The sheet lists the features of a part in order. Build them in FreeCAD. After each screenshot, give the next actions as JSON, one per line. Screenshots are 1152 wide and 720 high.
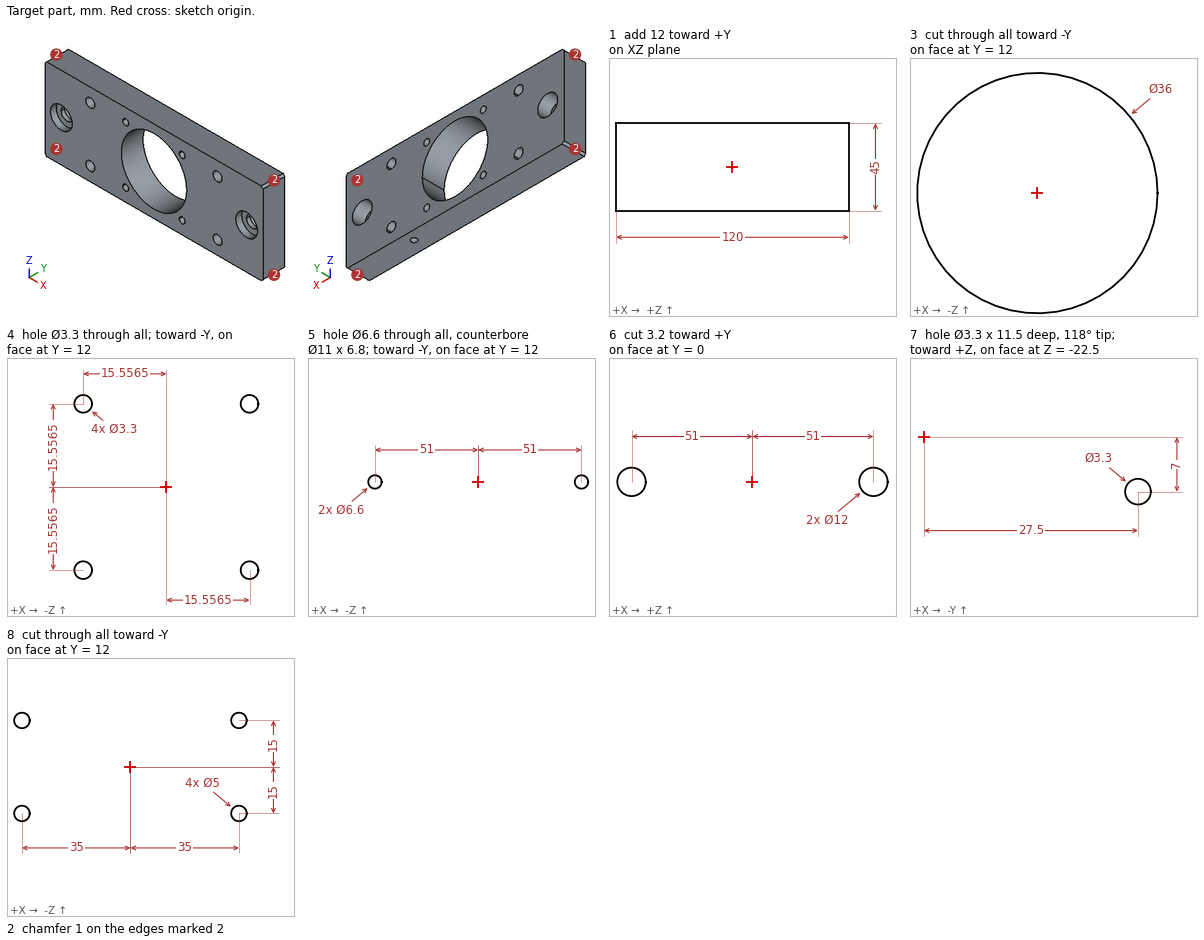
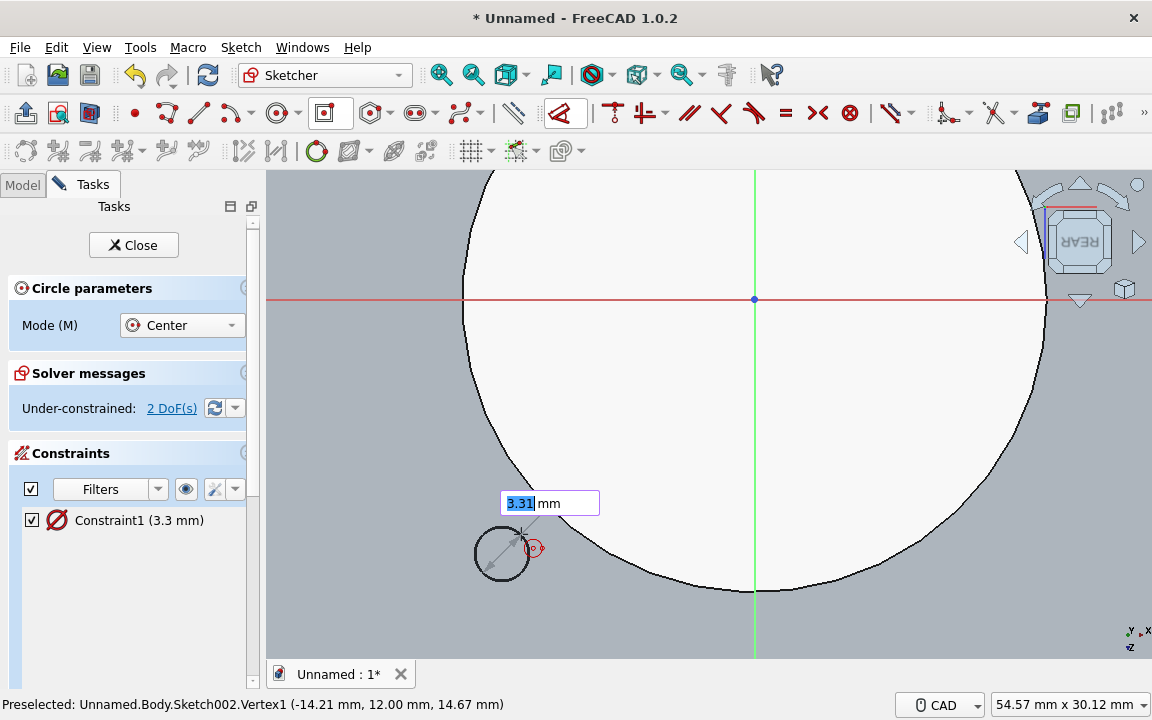
{"action": "type", "text": "3.3"}
{"action": "key", "text": "Return"}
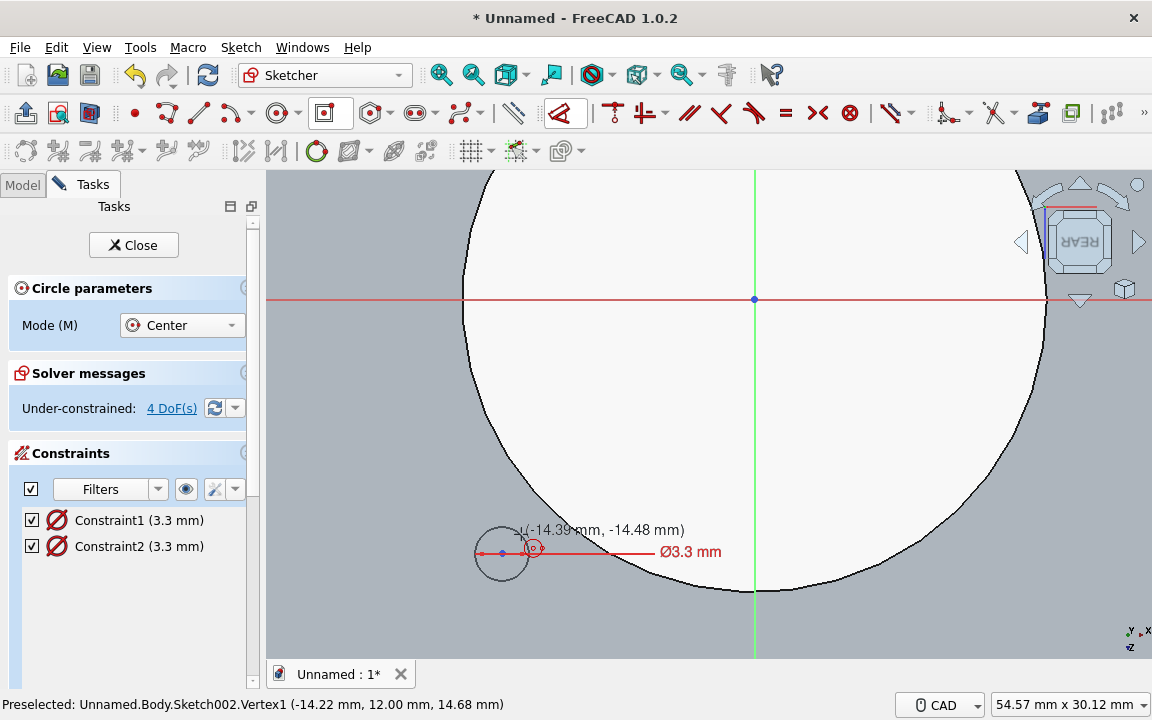
{"action": "scroll", "coordinate": [502, 554], "scroll_direction": "down", "scroll_amount": 3}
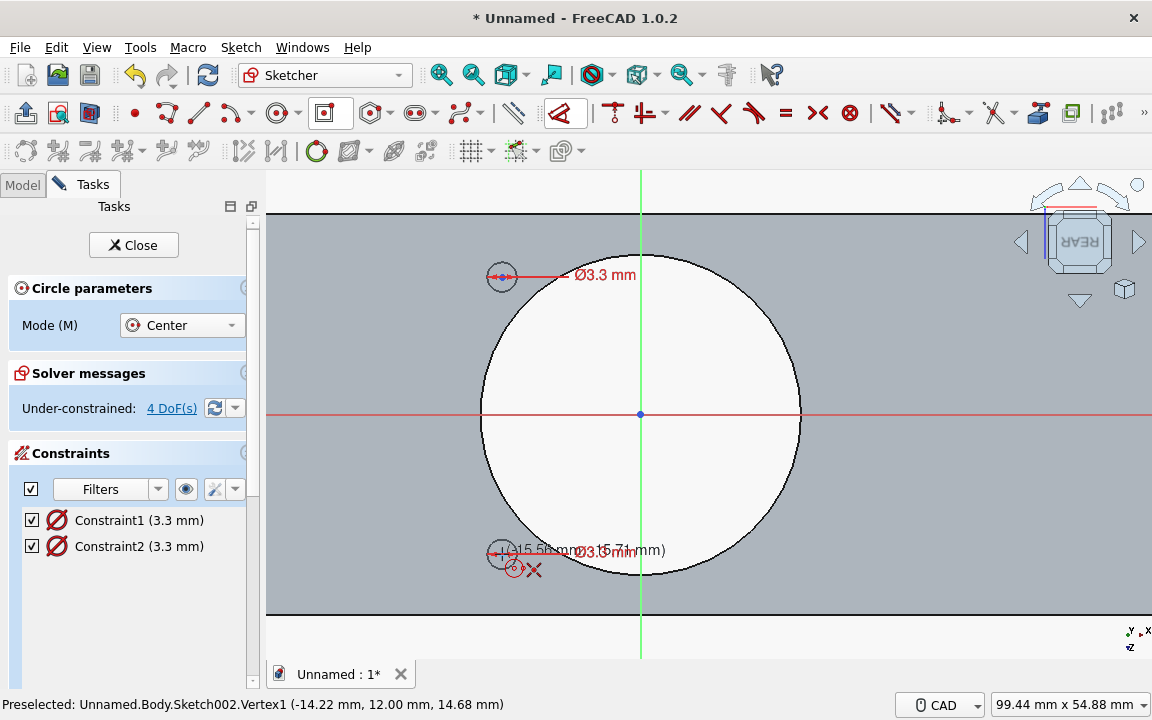
{"action": "scroll", "coordinate": [779, 554], "scroll_direction": "up", "scroll_amount": 3}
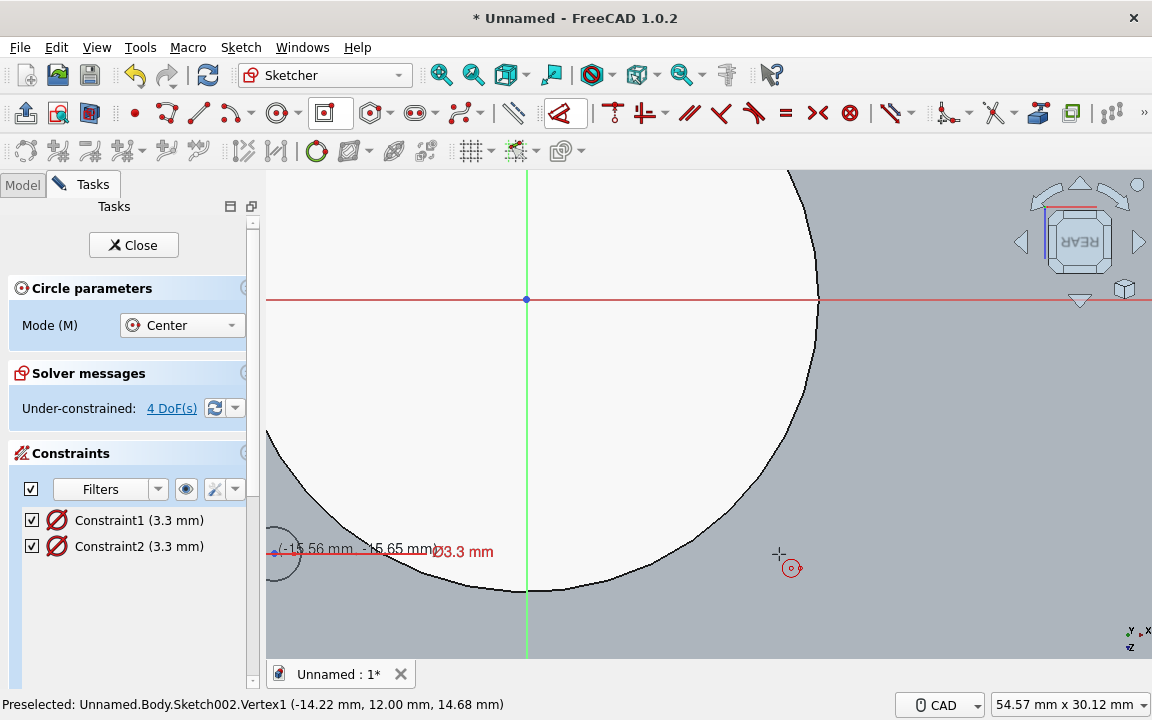
{"action": "left_click", "coordinate": [779, 553]}
{"action": "mouse_move", "coordinate": [798, 534]}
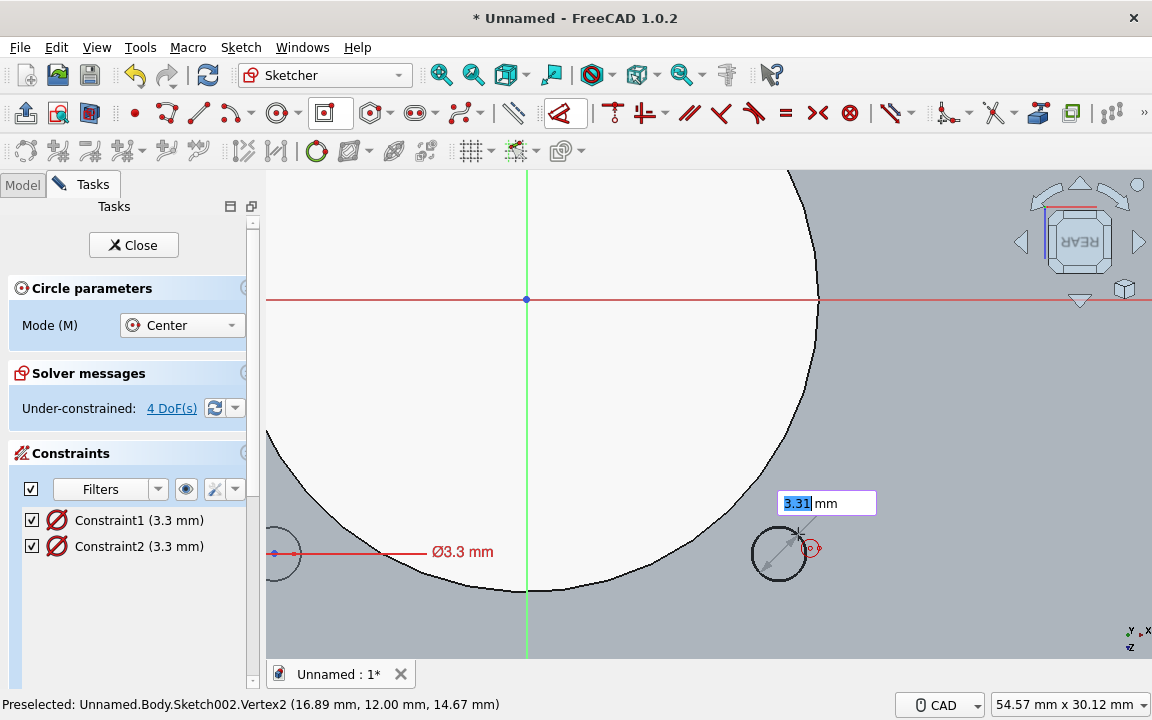
{"action": "type", "text": "3.3"}
{"action": "key", "text": "Return"}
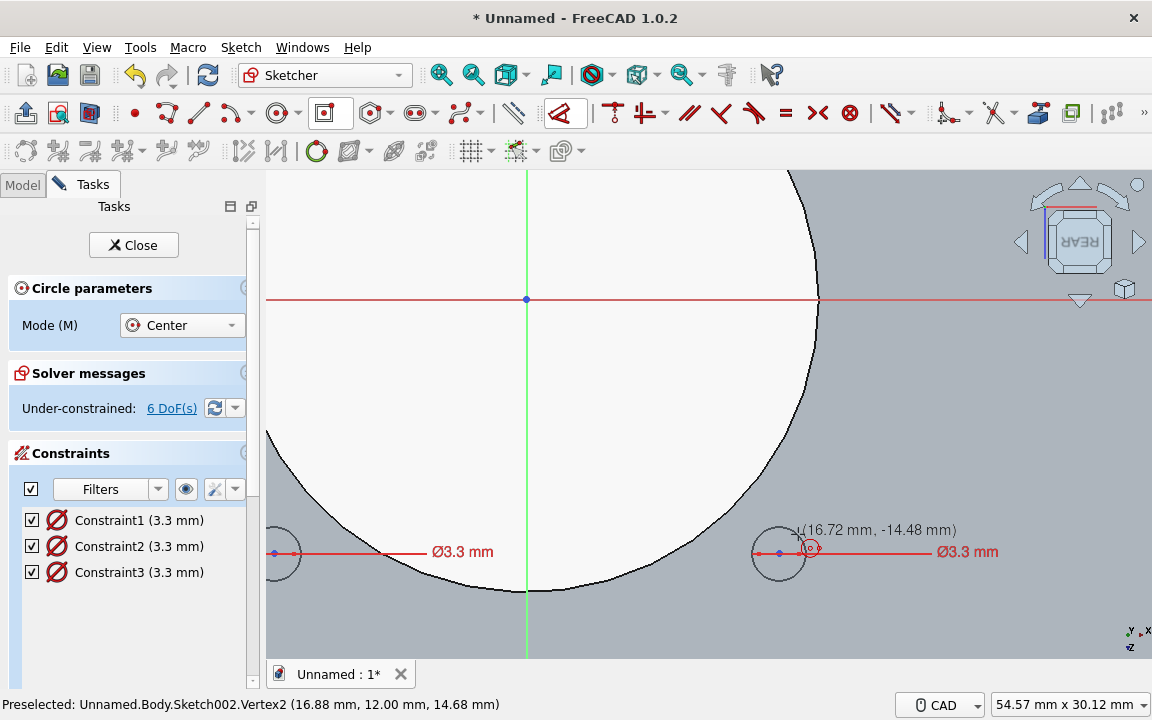
{"action": "scroll", "coordinate": [779, 554], "scroll_direction": "down", "scroll_amount": 3}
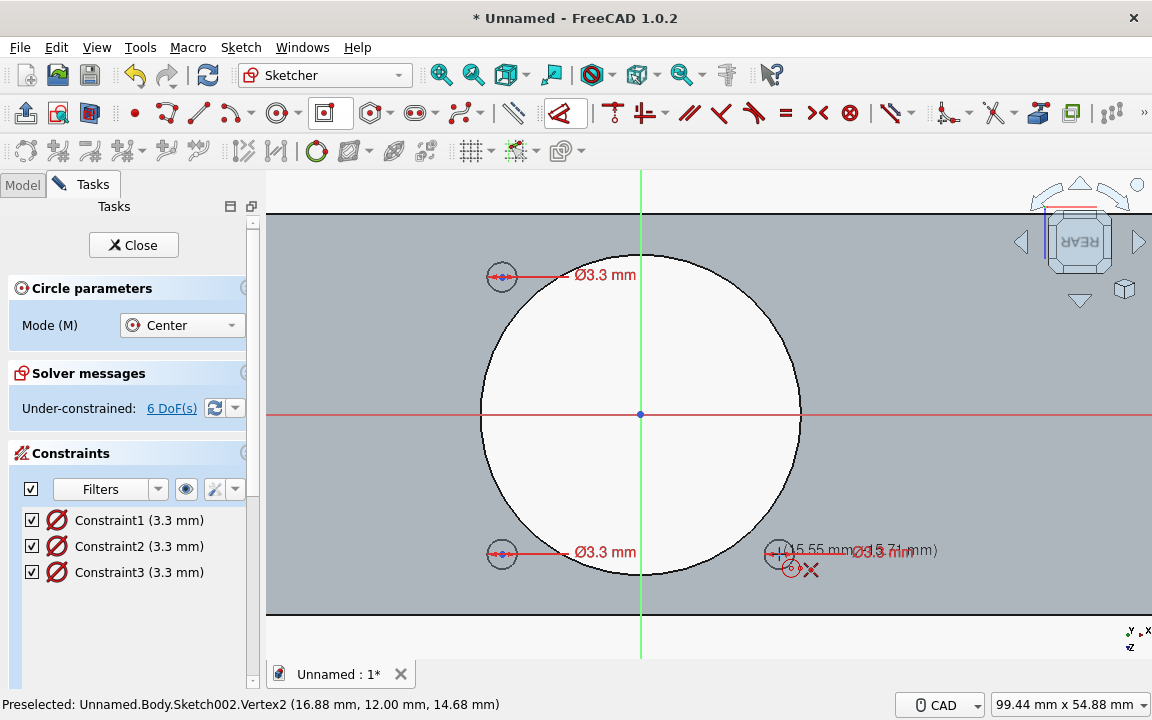
{"action": "scroll", "coordinate": [779, 276], "scroll_direction": "up", "scroll_amount": 3}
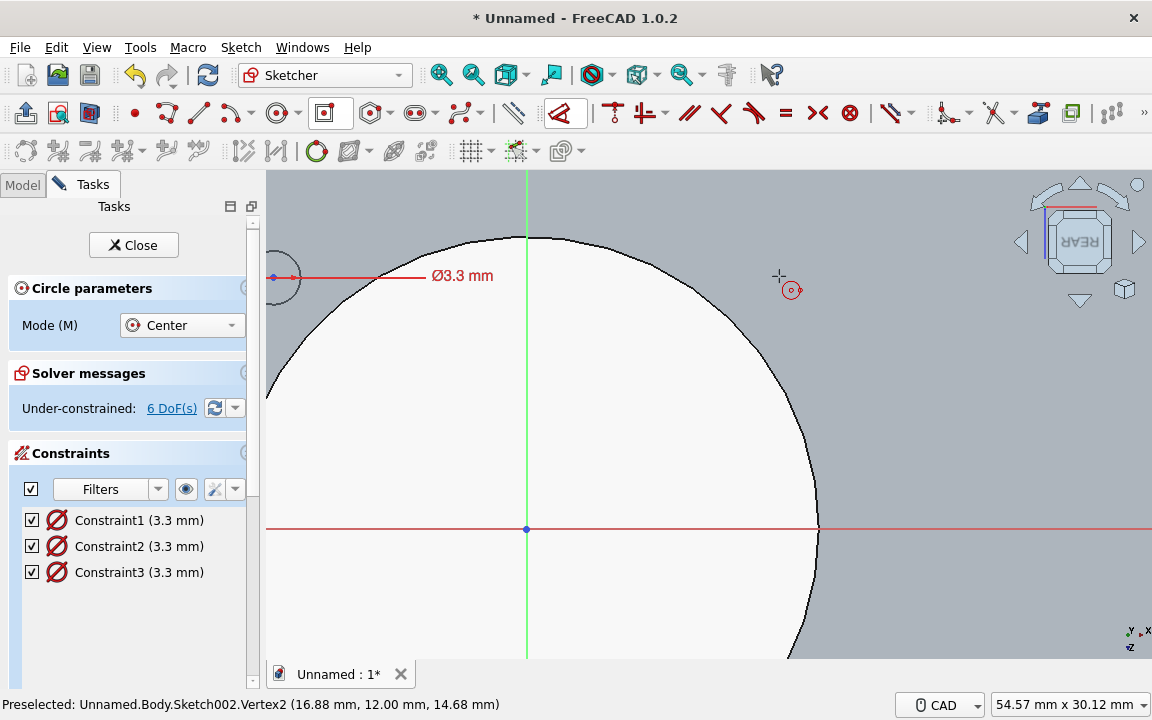
{"action": "left_click", "coordinate": [779, 276]}
{"action": "mouse_move", "coordinate": [798, 258]}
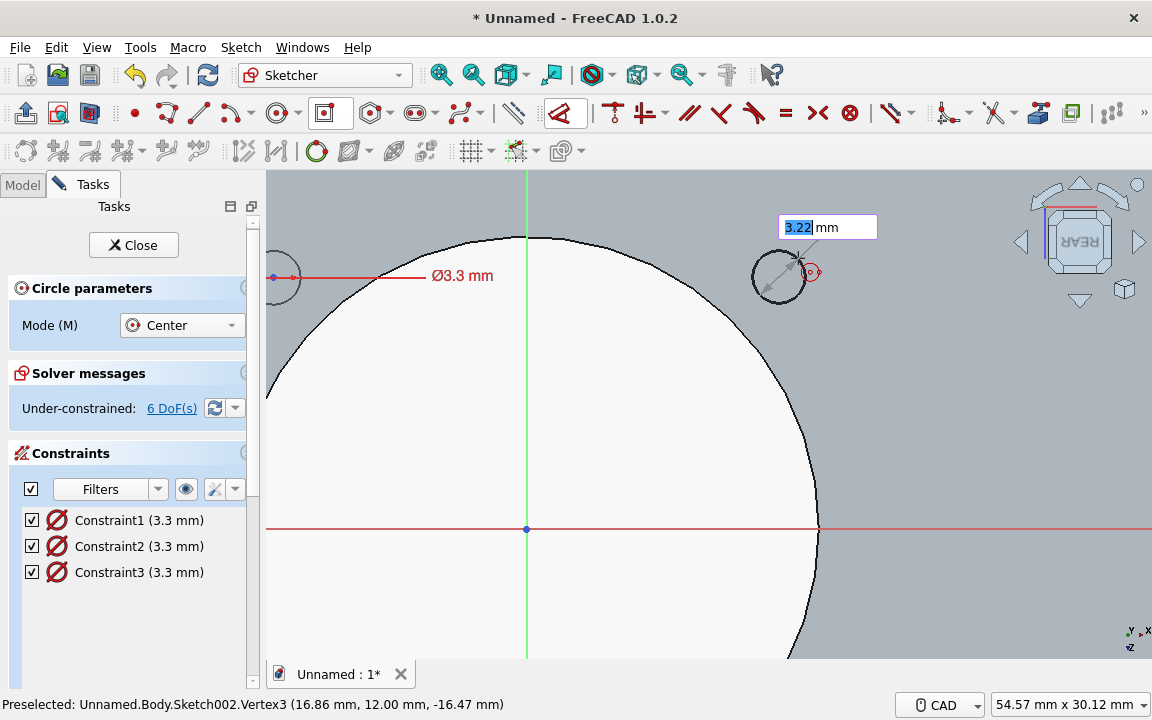
{"action": "type", "text": "3.3"}
{"action": "key", "text": "Return"}
{"action": "key", "text": "Escape"}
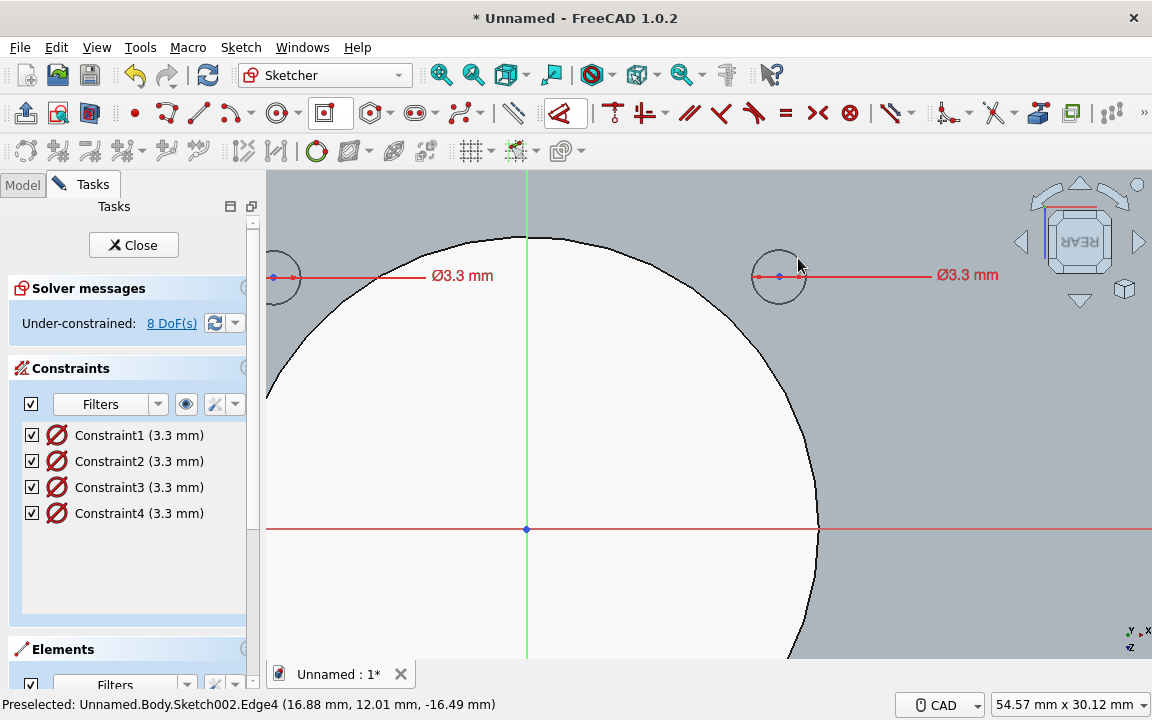
{"action": "scroll", "coordinate": [779, 275], "scroll_direction": "down", "scroll_amount": 3}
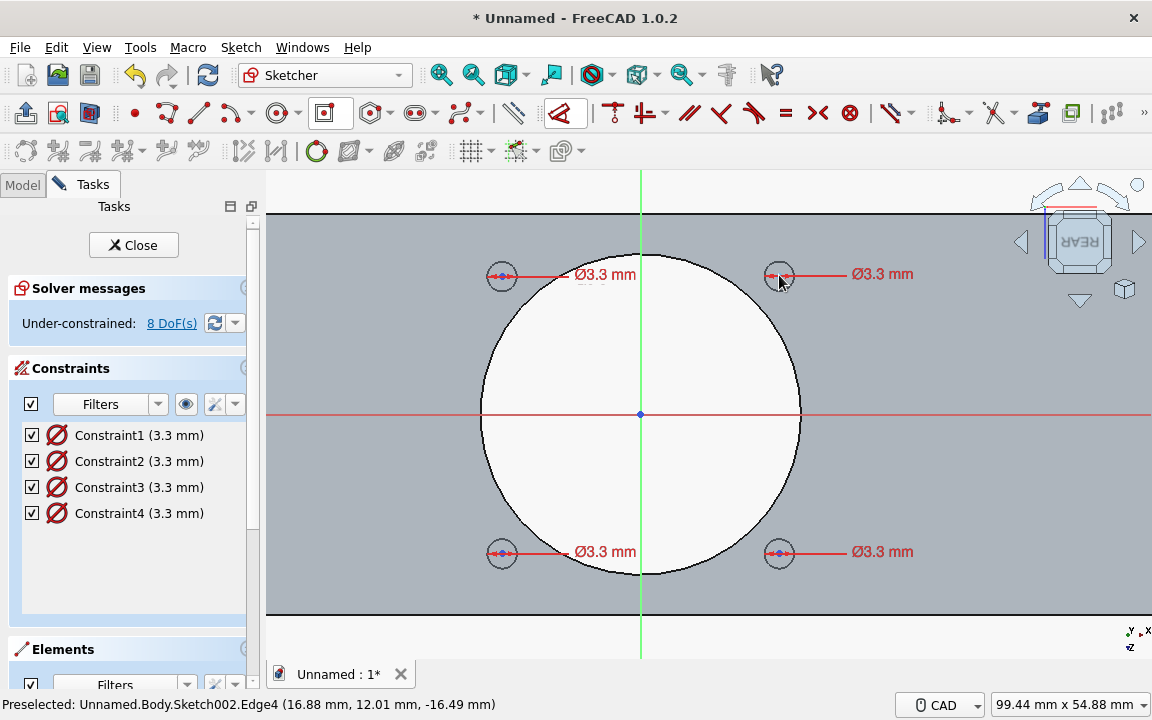
{"action": "left_click", "coordinate": [502, 277]}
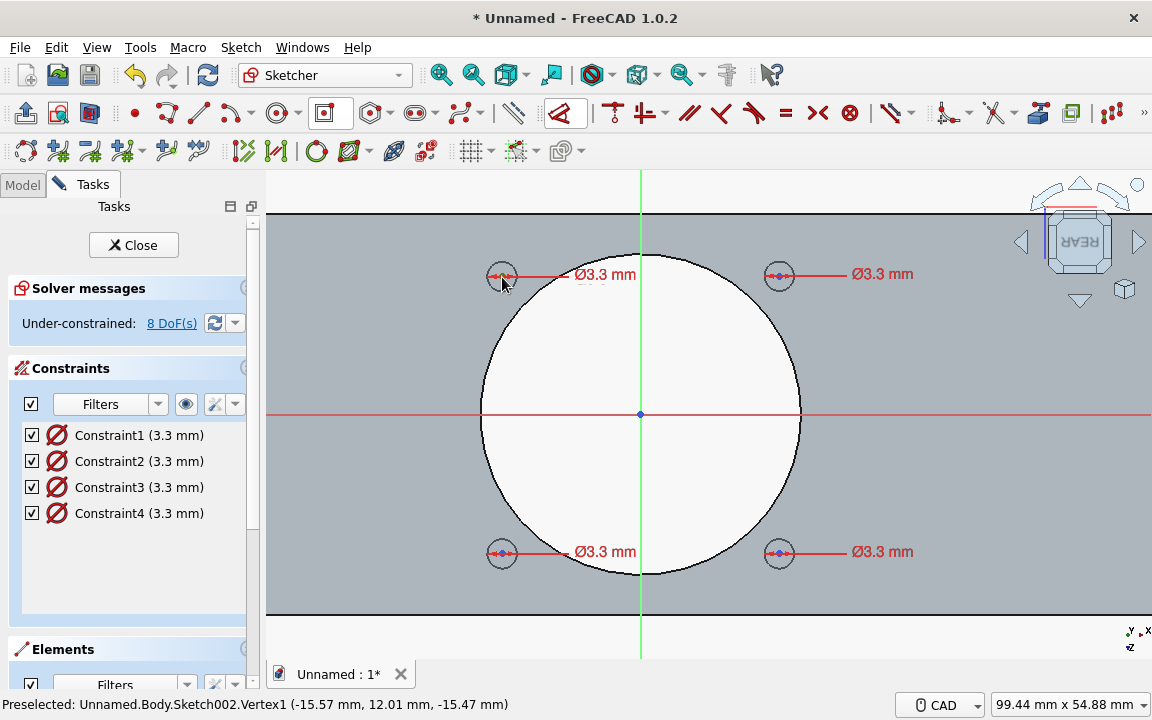
{"action": "left_click", "coordinate": [502, 554]}